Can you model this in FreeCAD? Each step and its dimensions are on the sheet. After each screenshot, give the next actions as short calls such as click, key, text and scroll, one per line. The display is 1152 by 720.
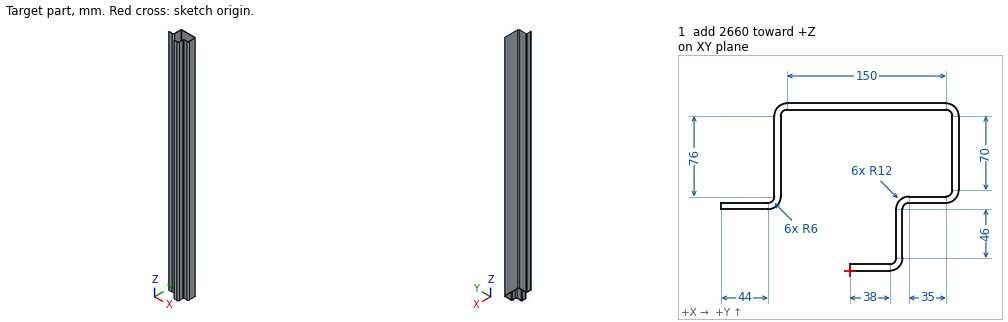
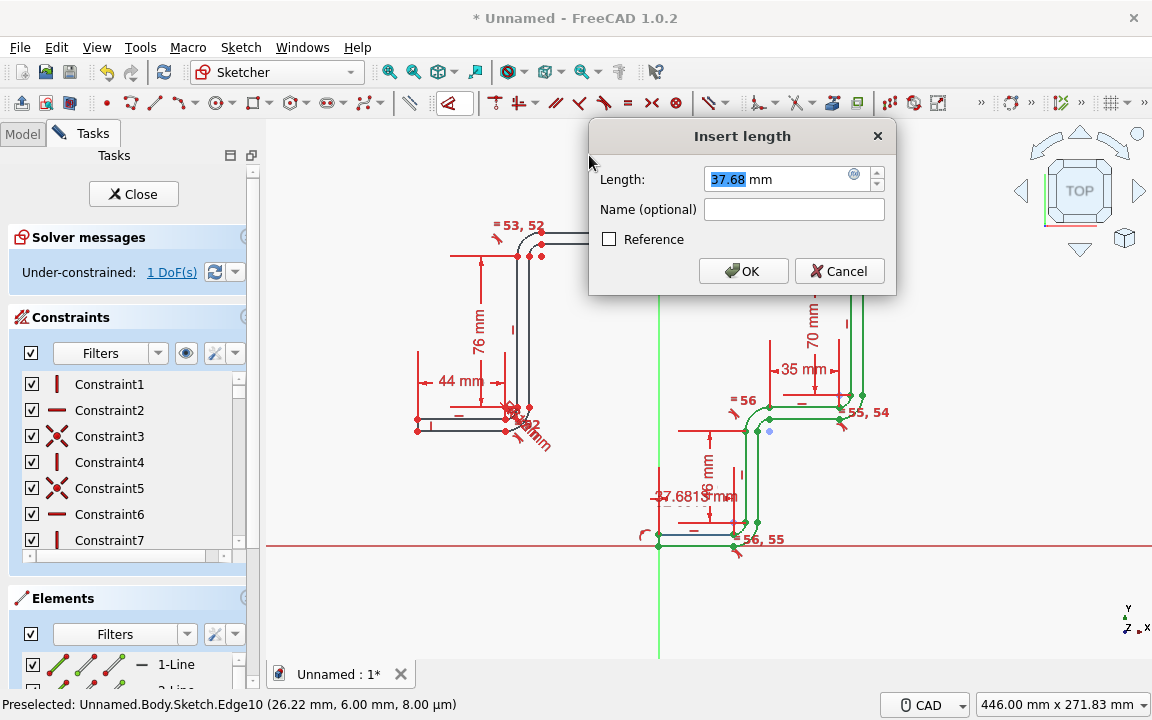
text(38)
key(Return)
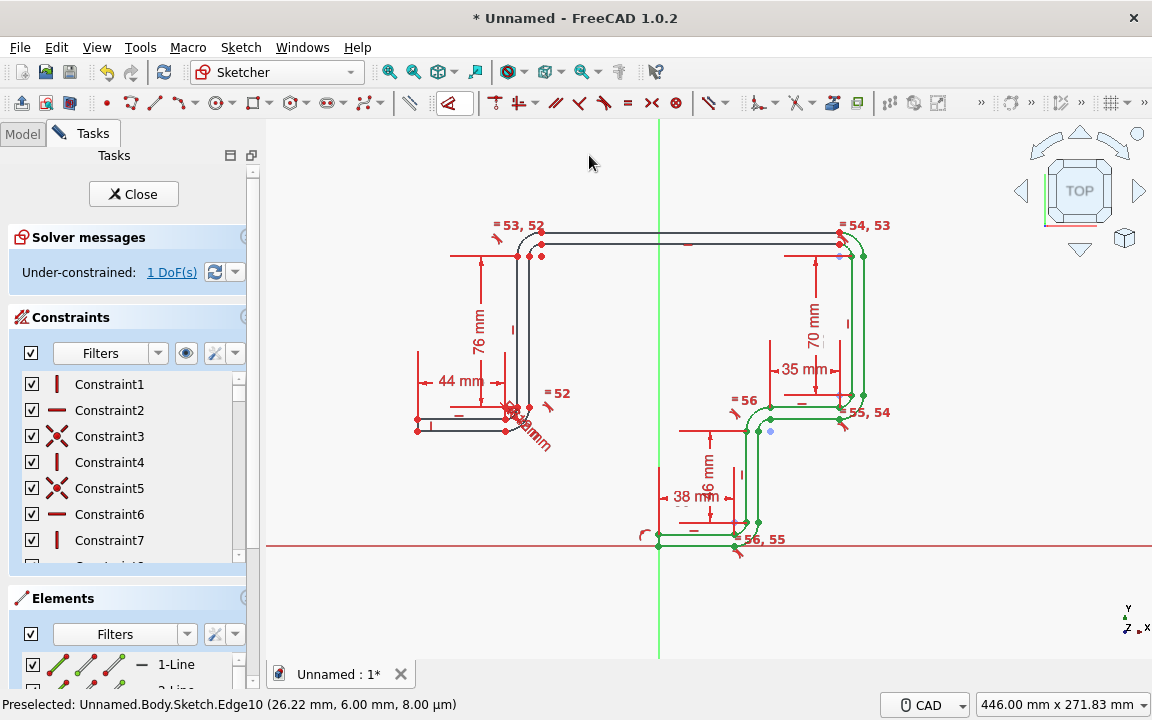
click(631, 244)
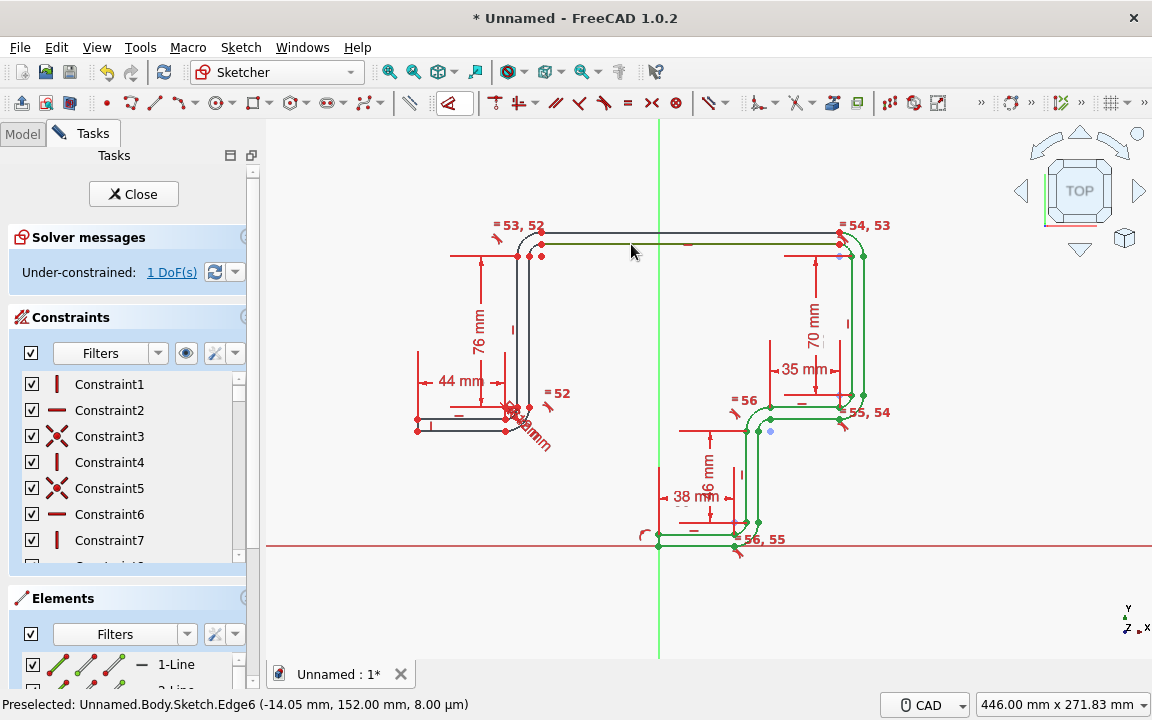
key(l)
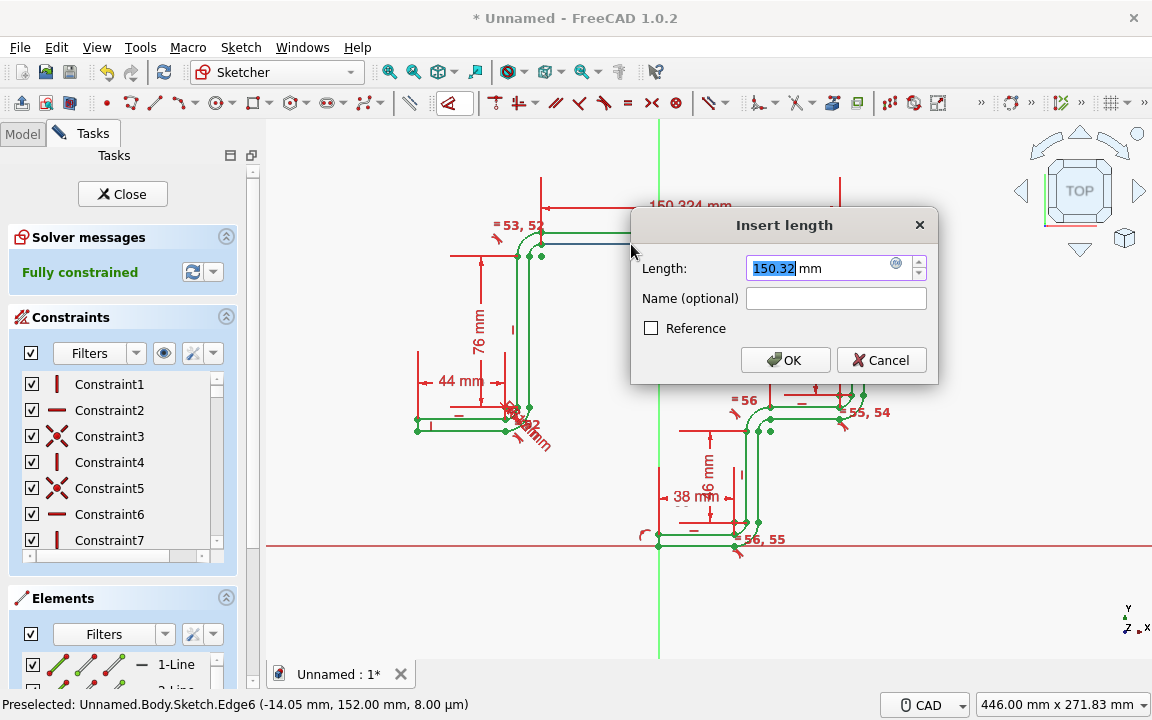
text(150)
key(Return)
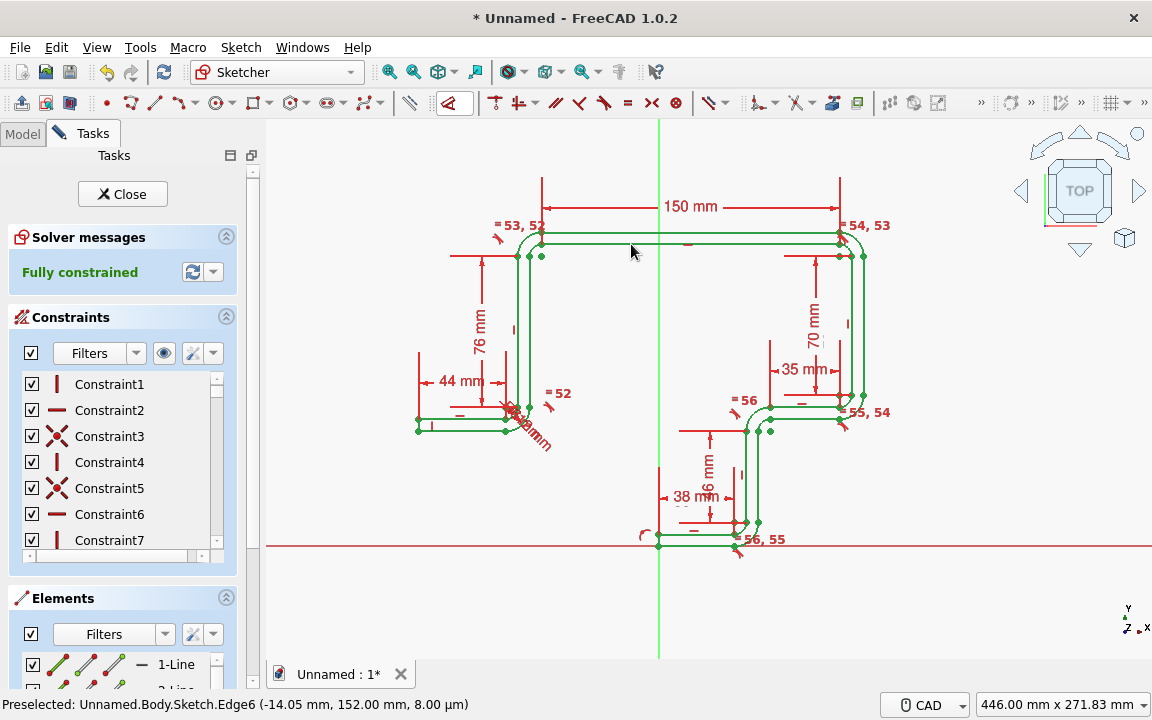
click(123, 194)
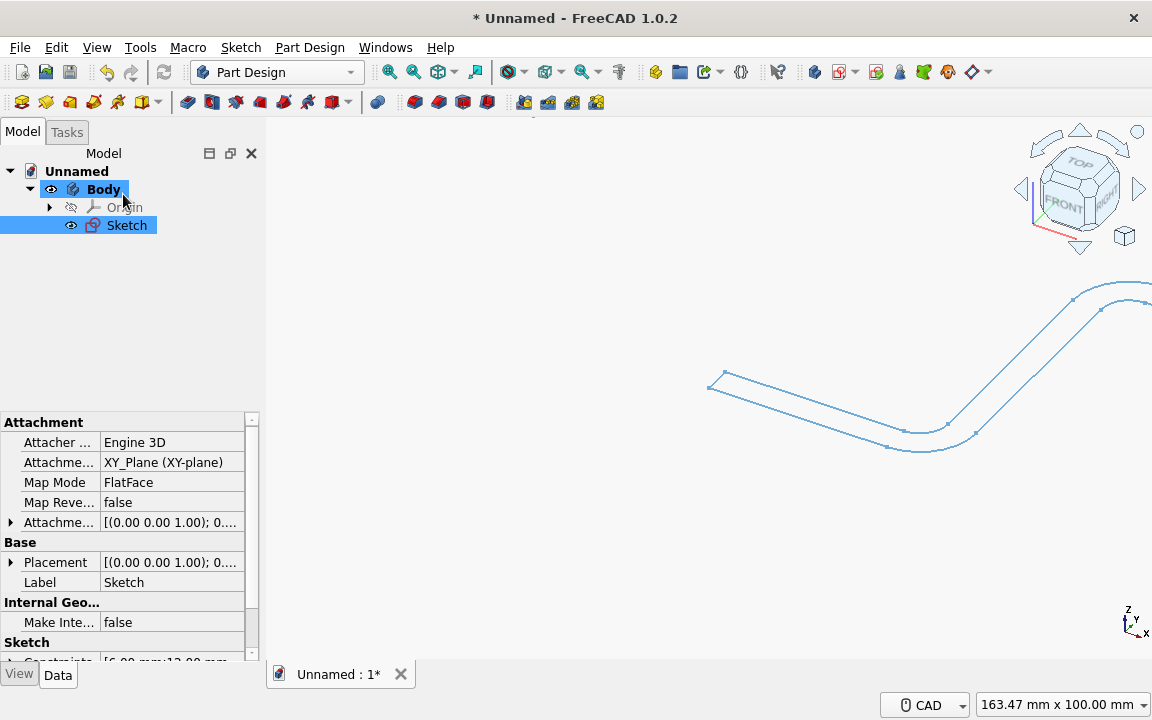
click(22, 102)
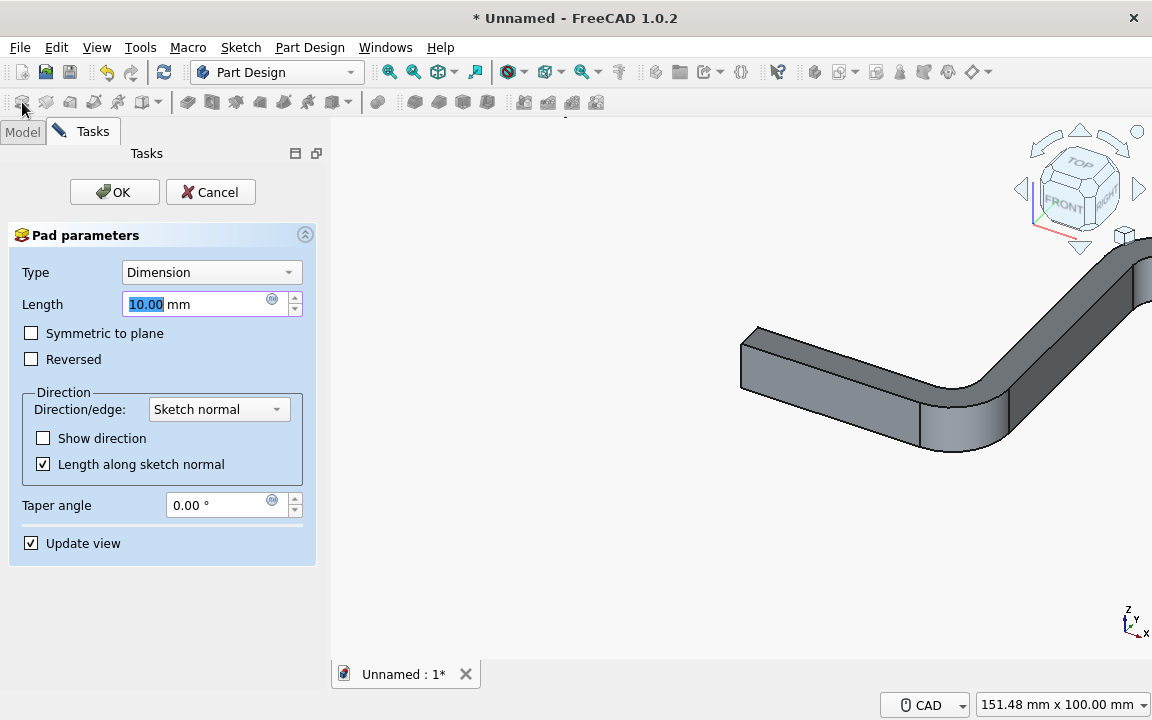
text(2660)
key(Tab)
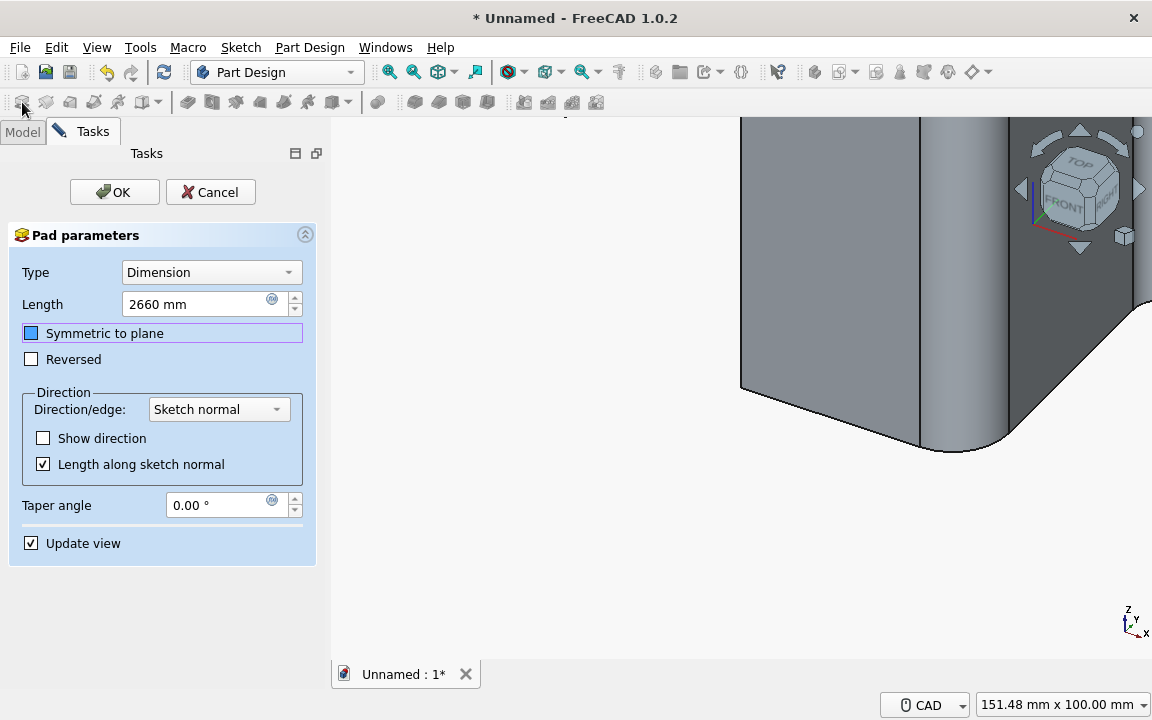
click(115, 192)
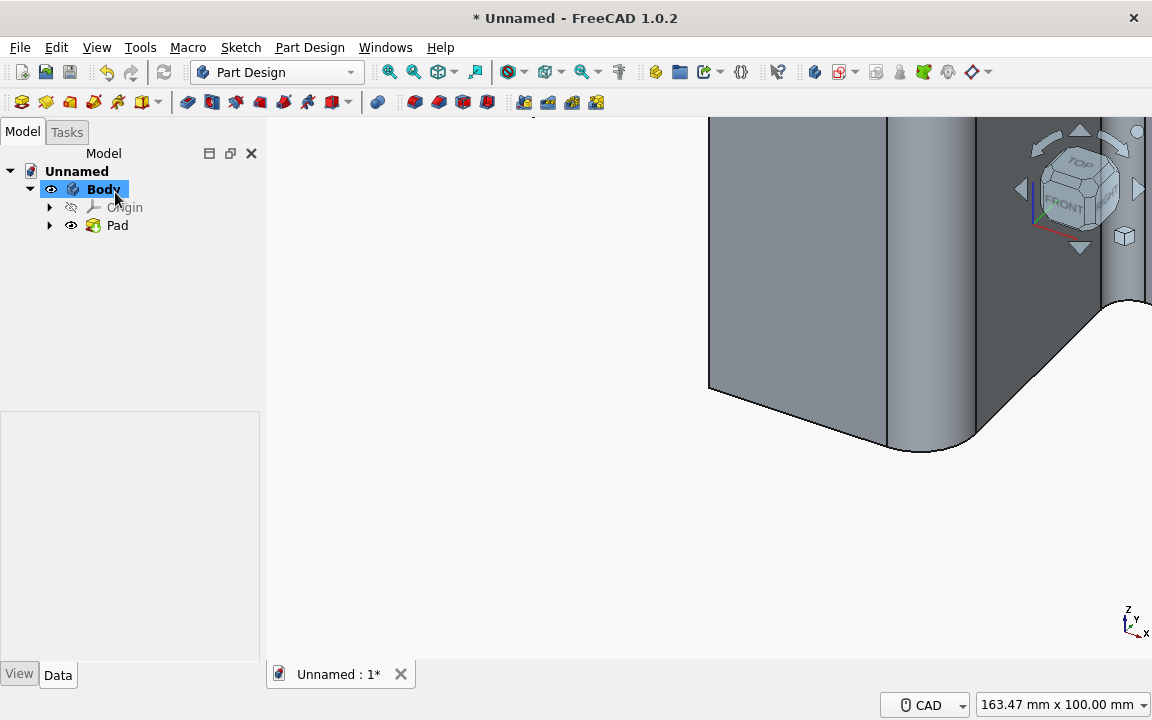
key(0)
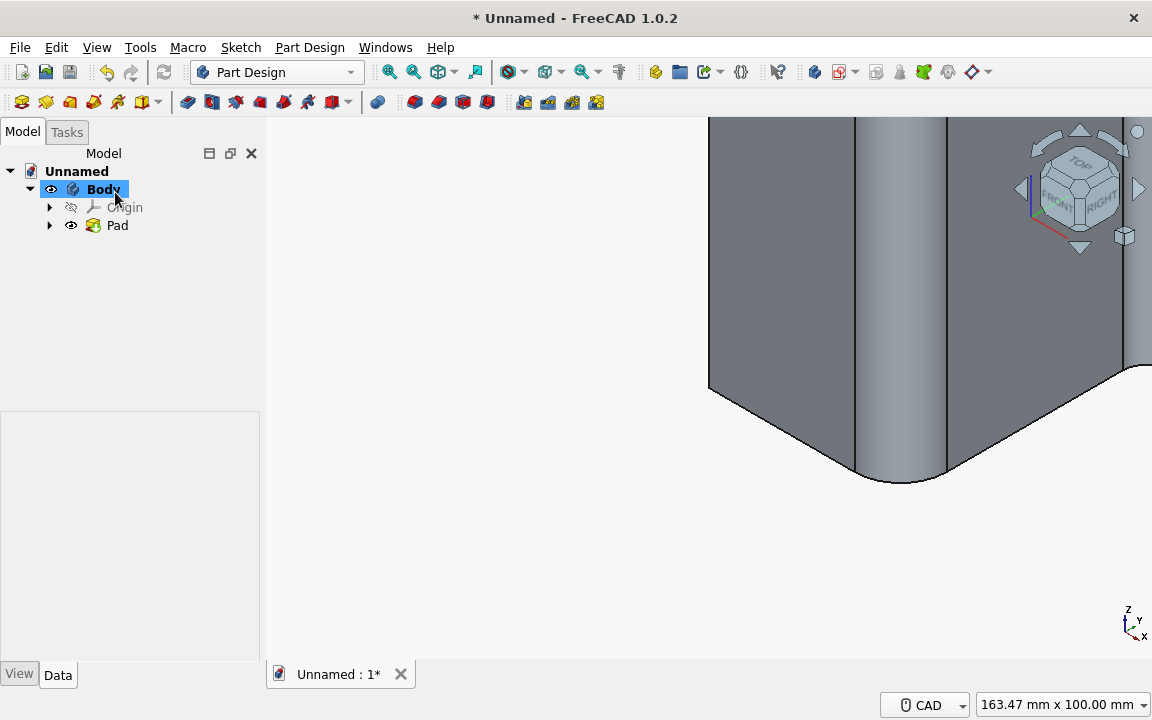
key(v)
key(f)